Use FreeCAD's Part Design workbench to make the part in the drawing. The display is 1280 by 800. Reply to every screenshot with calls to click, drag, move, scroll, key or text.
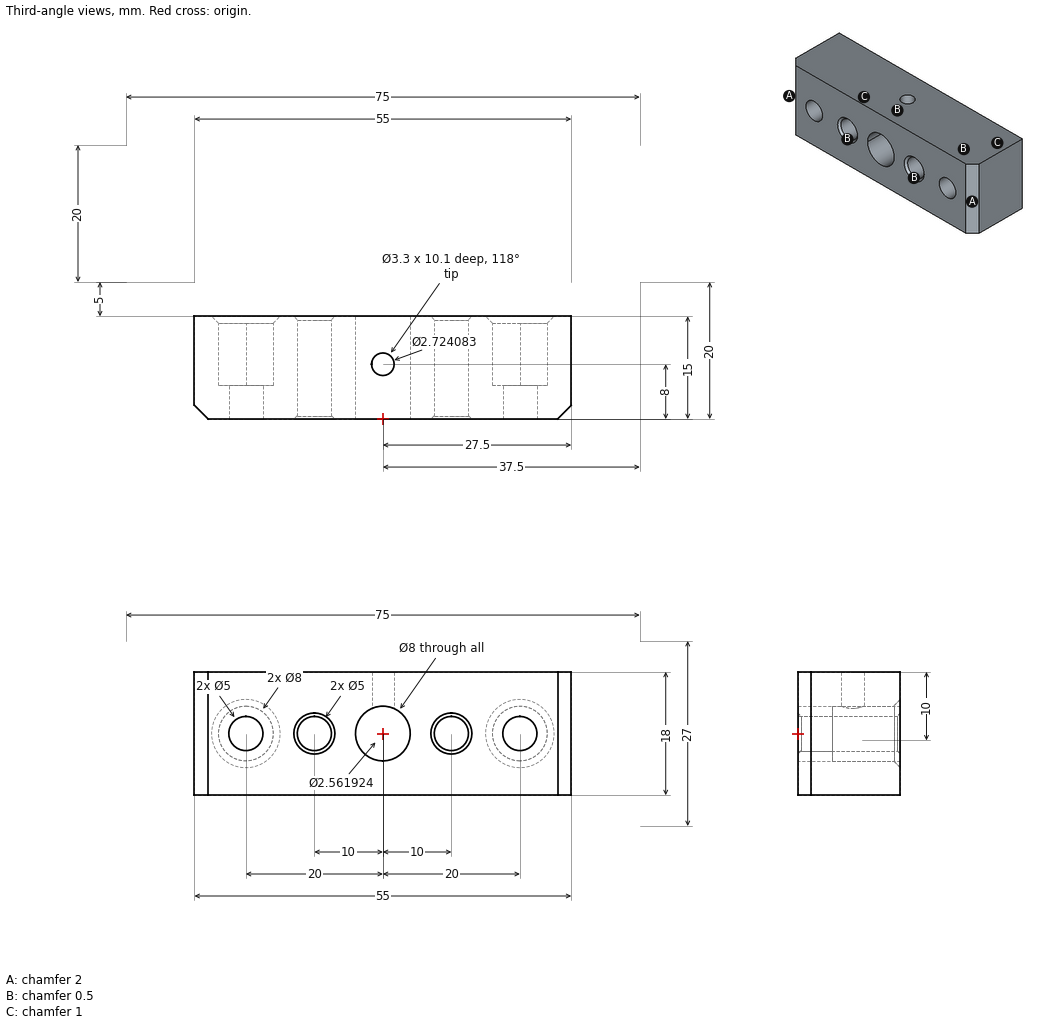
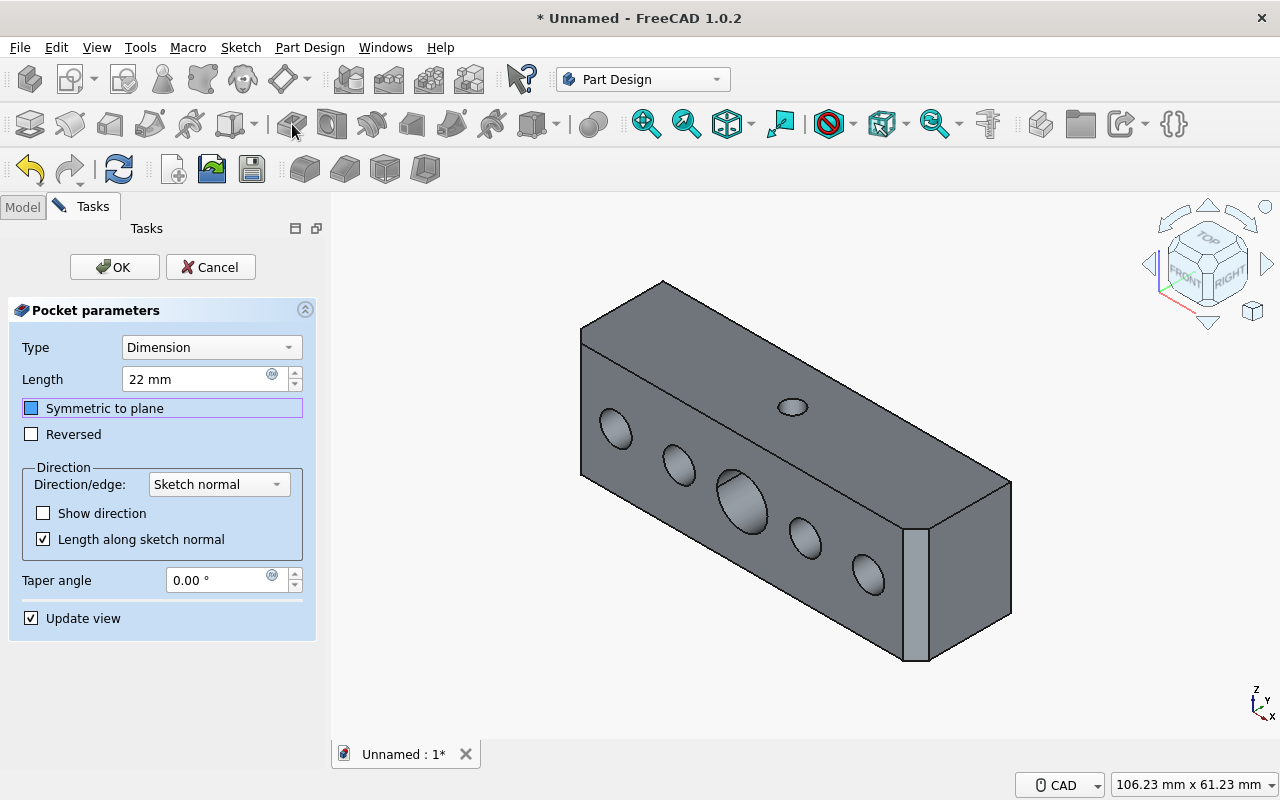
click(115, 267)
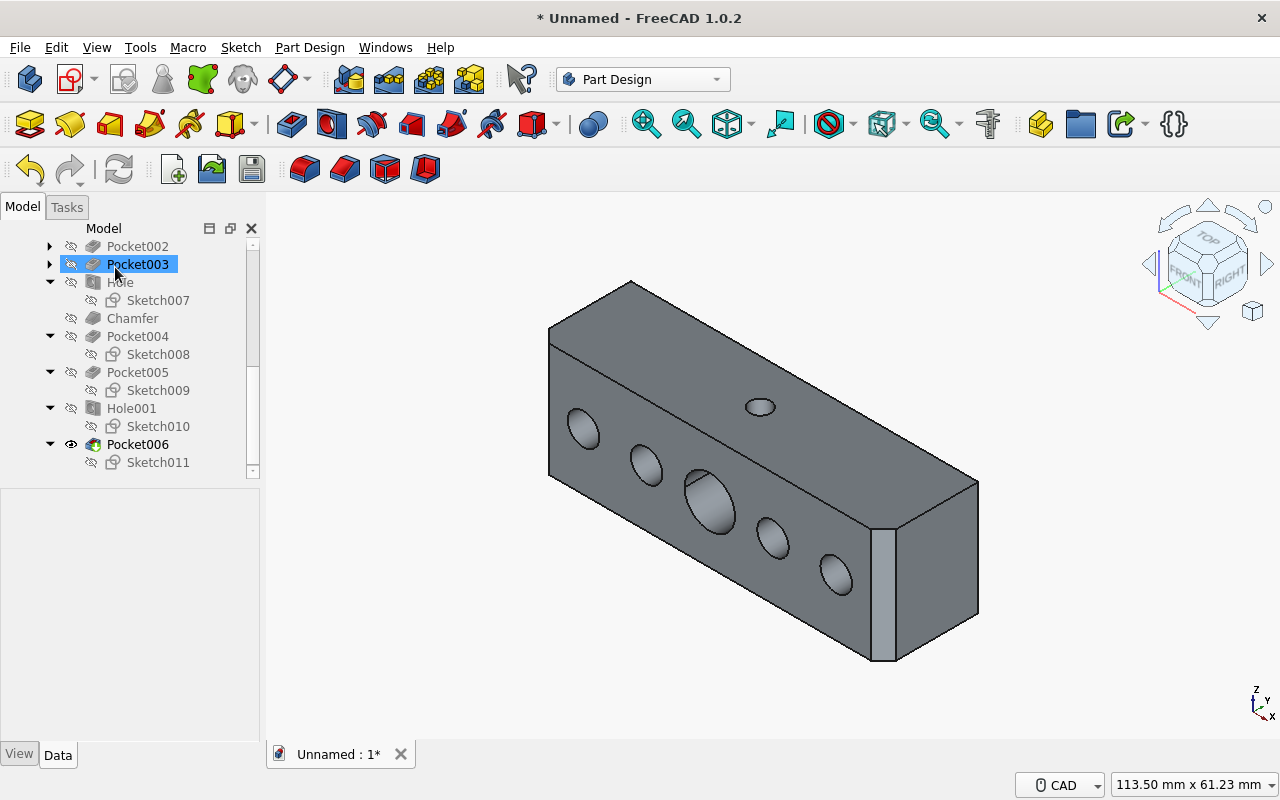
click(631, 455)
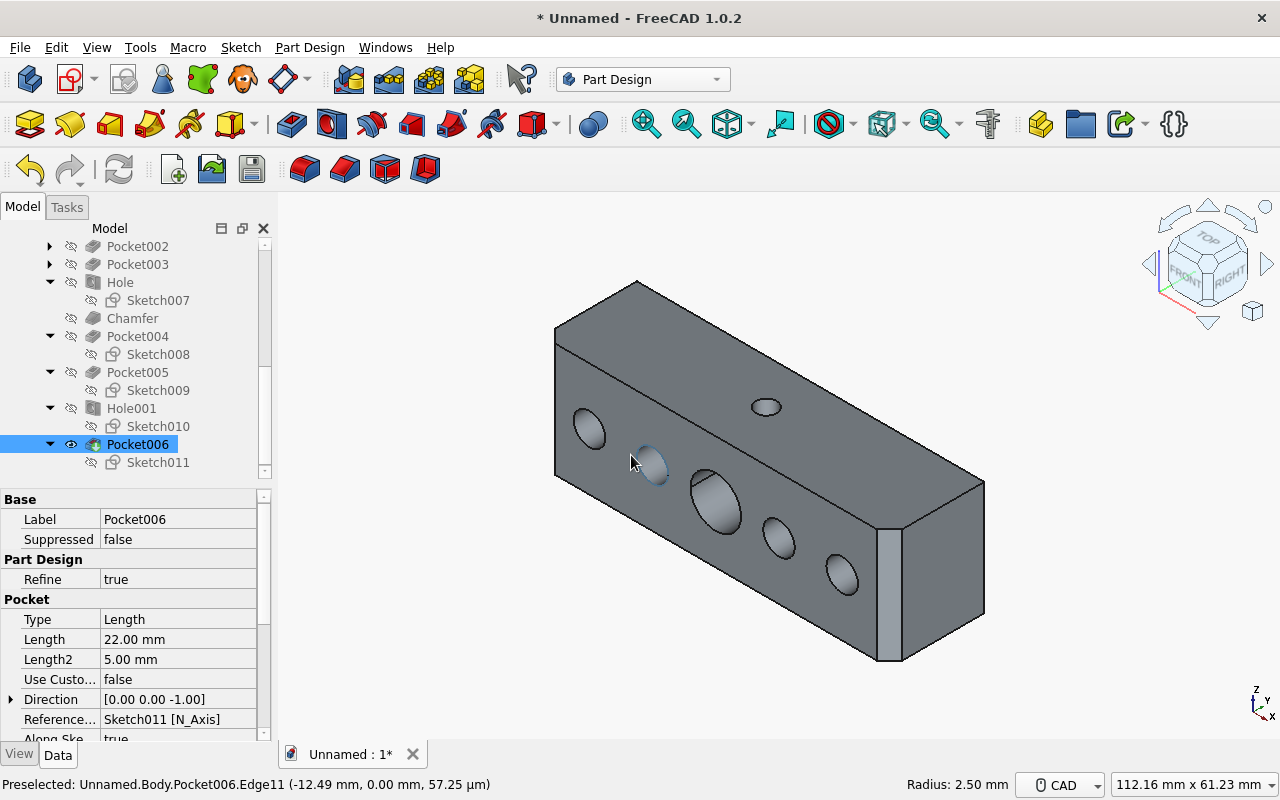
click(763, 528, ctrl)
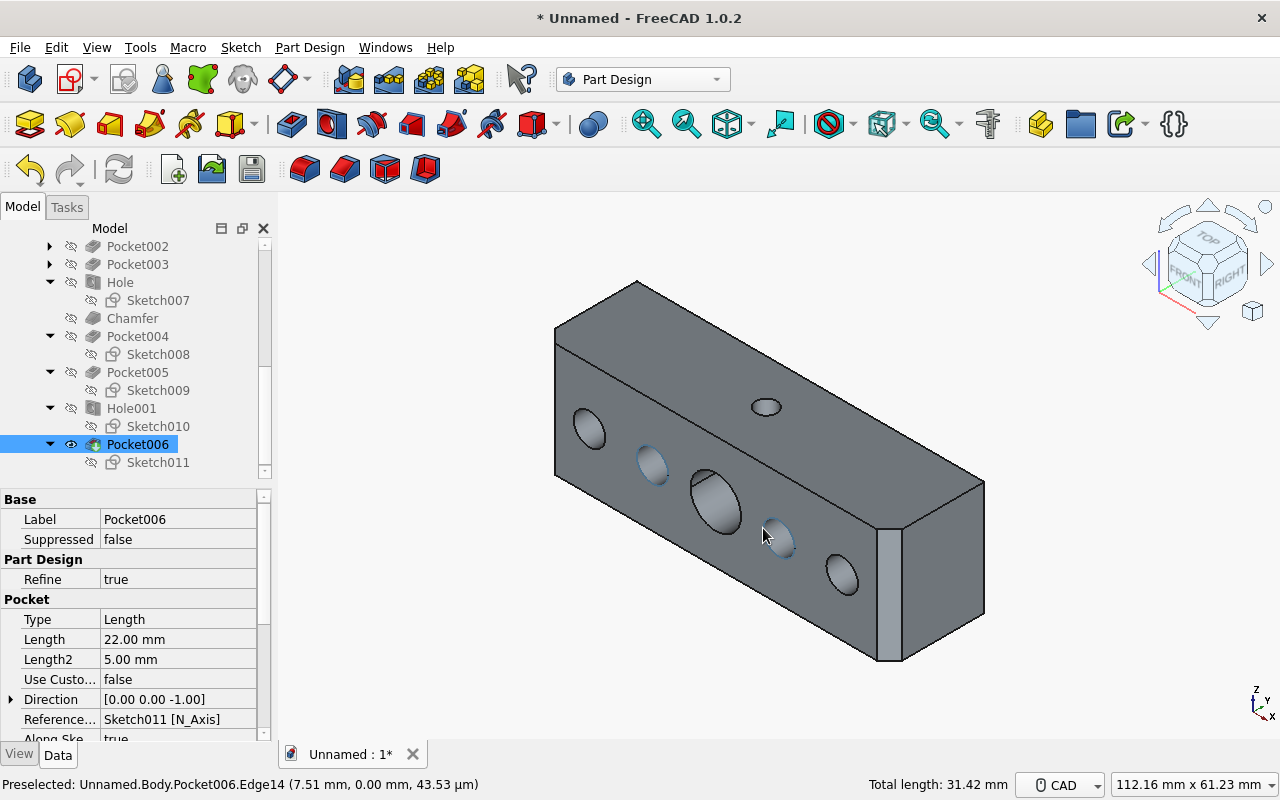
key(2)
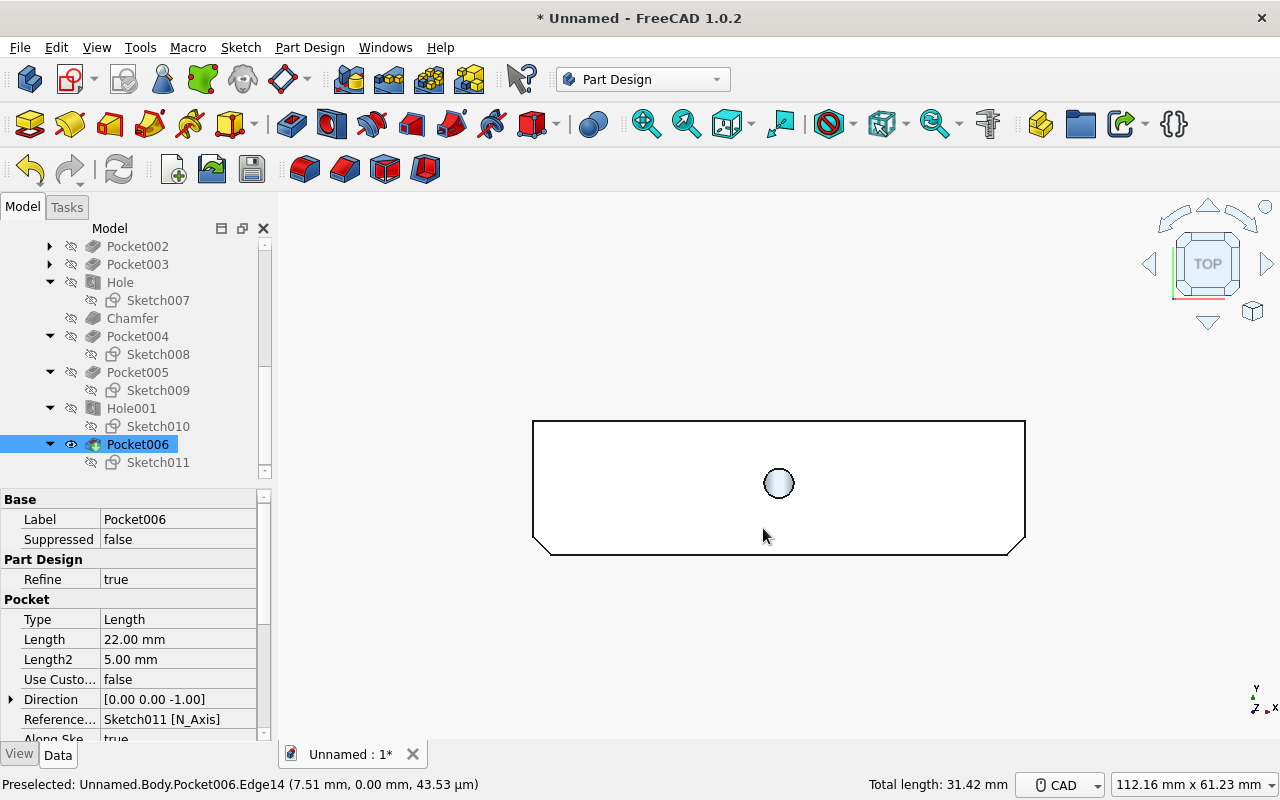
key(0)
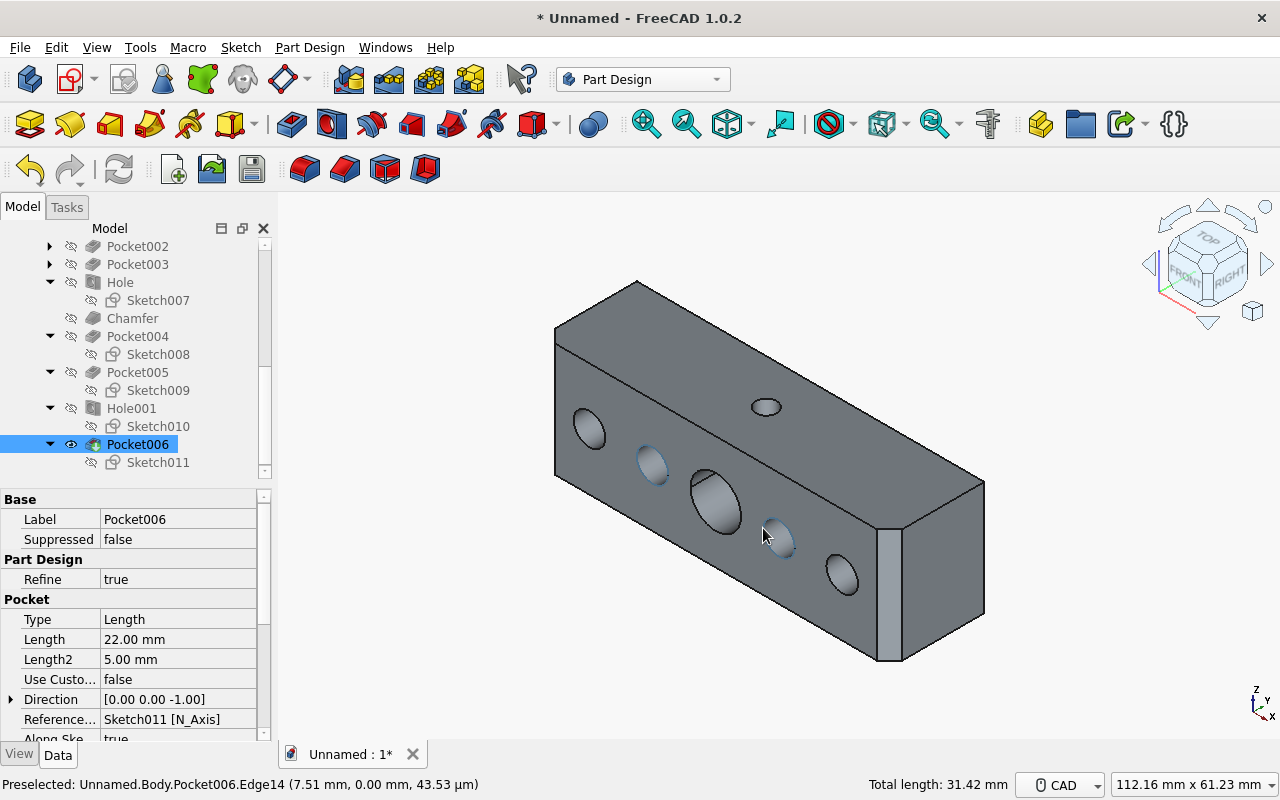
key(1)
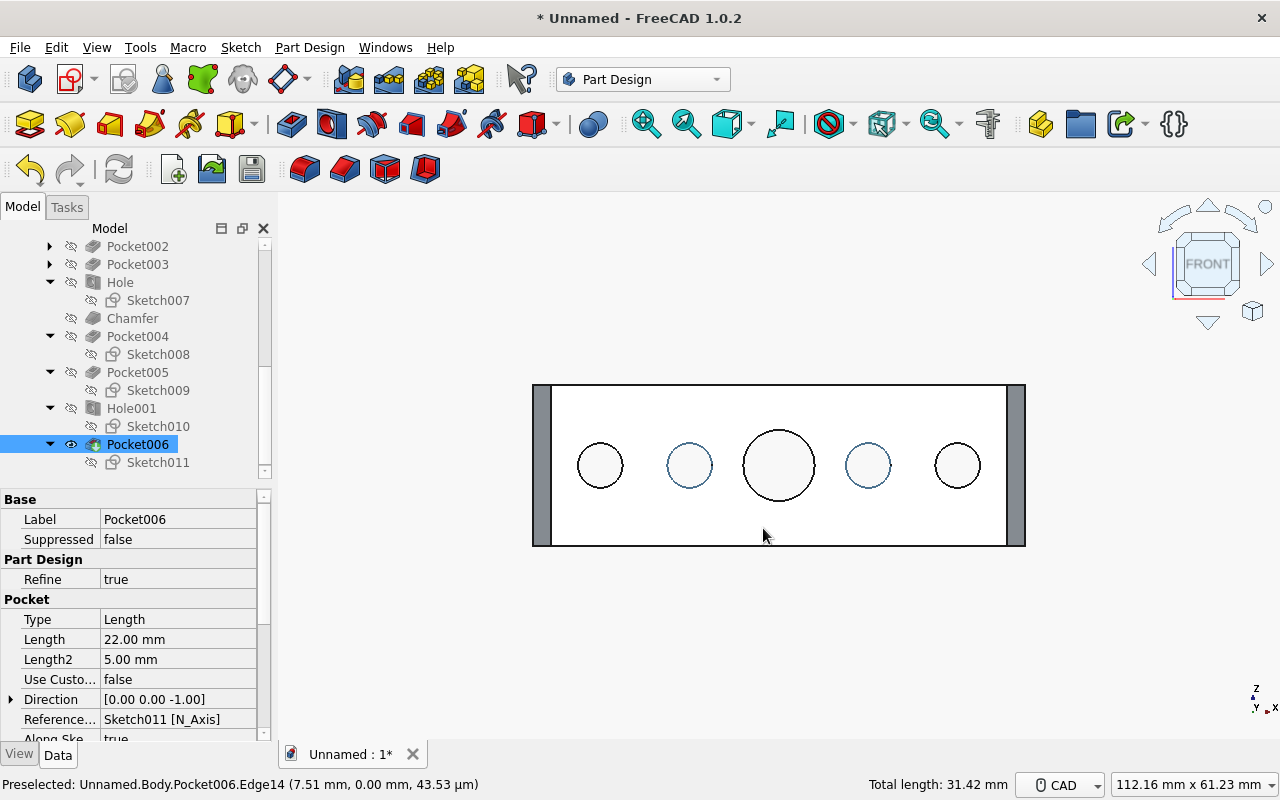
key(3)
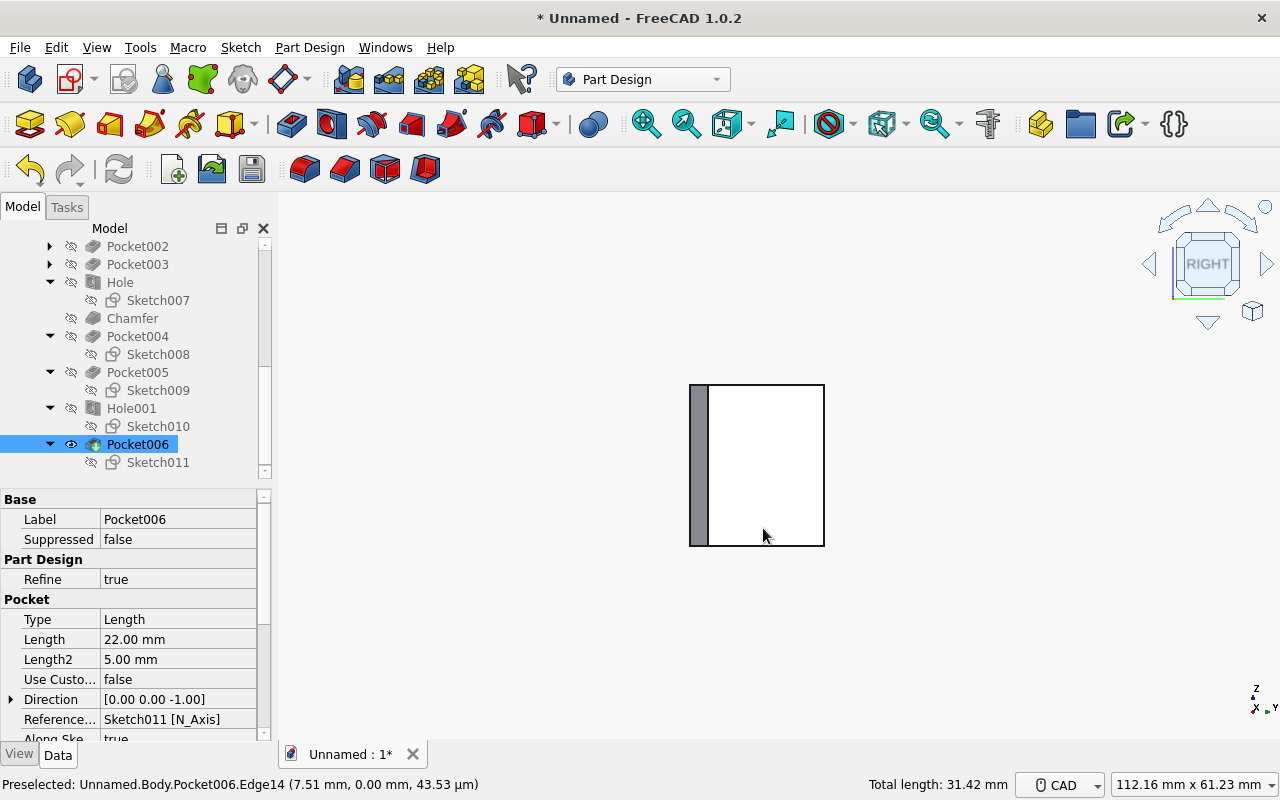
click(648, 124)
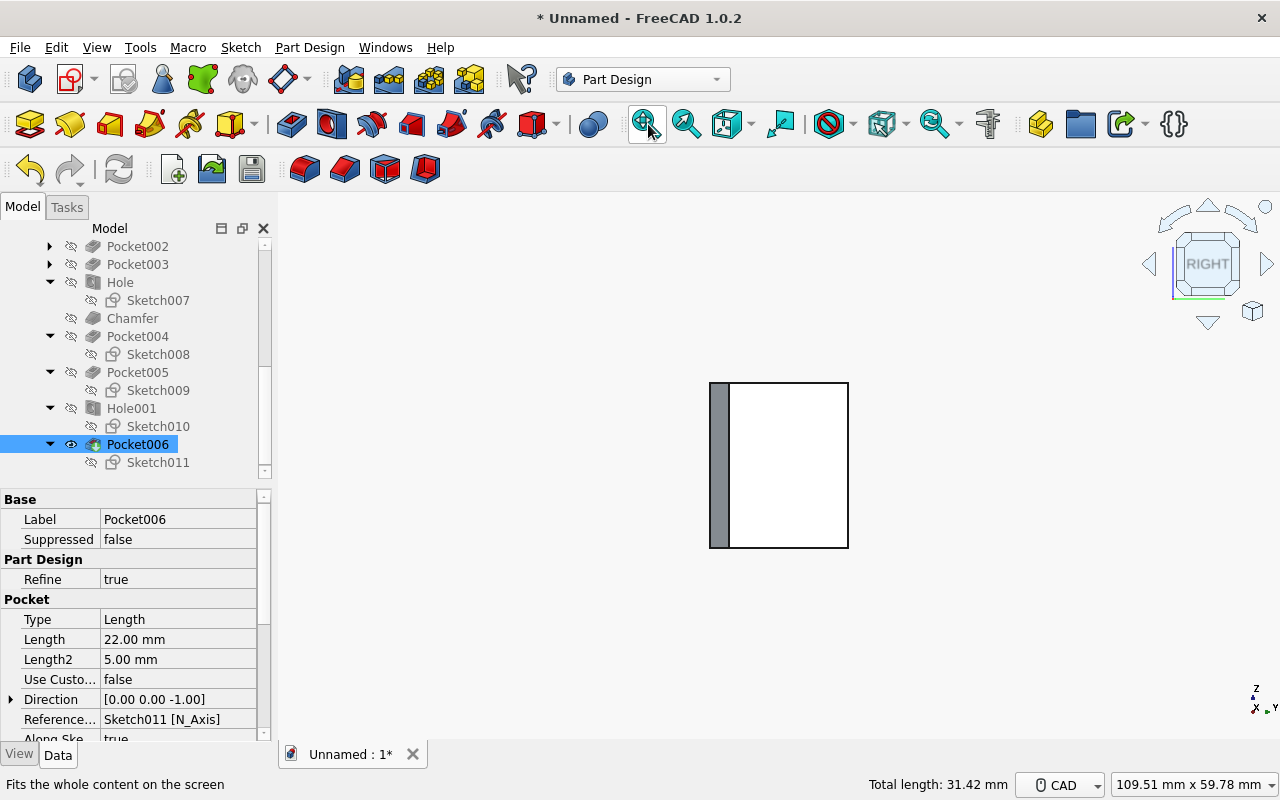
key(5)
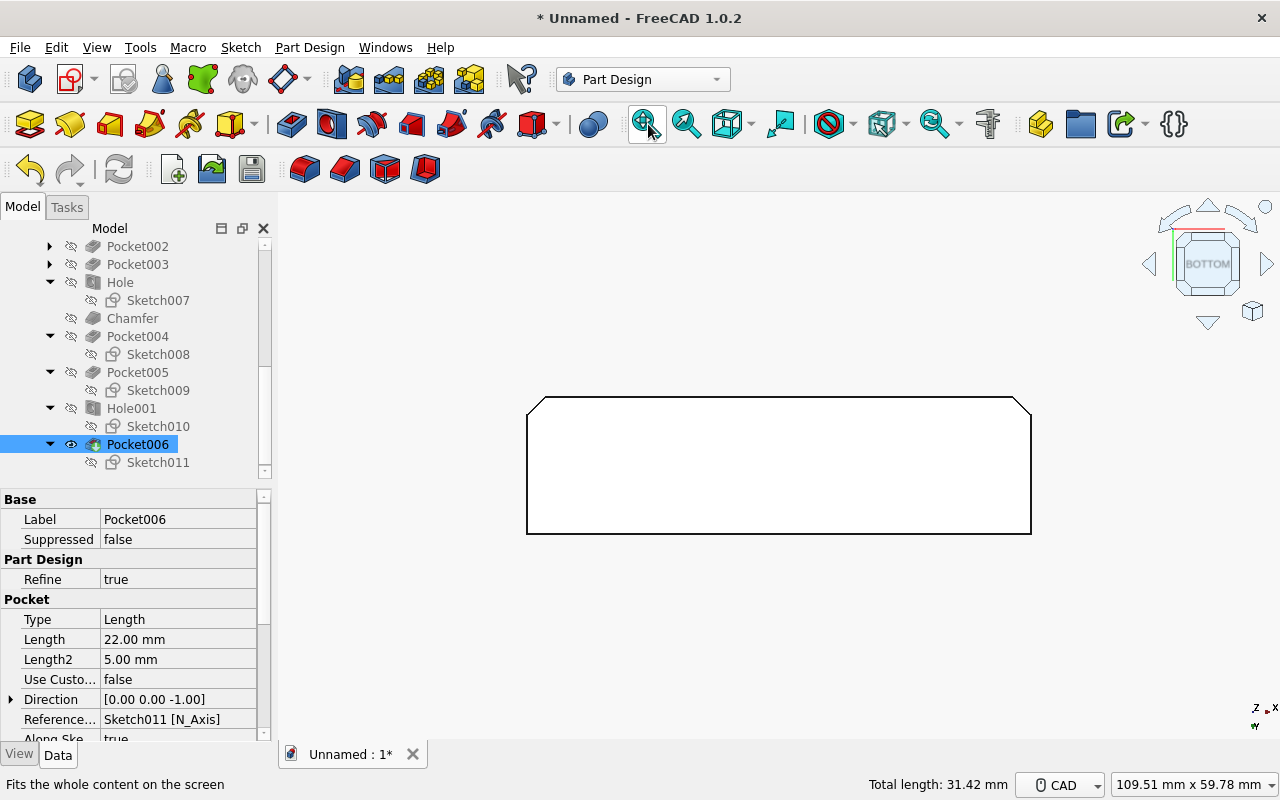
key(4)